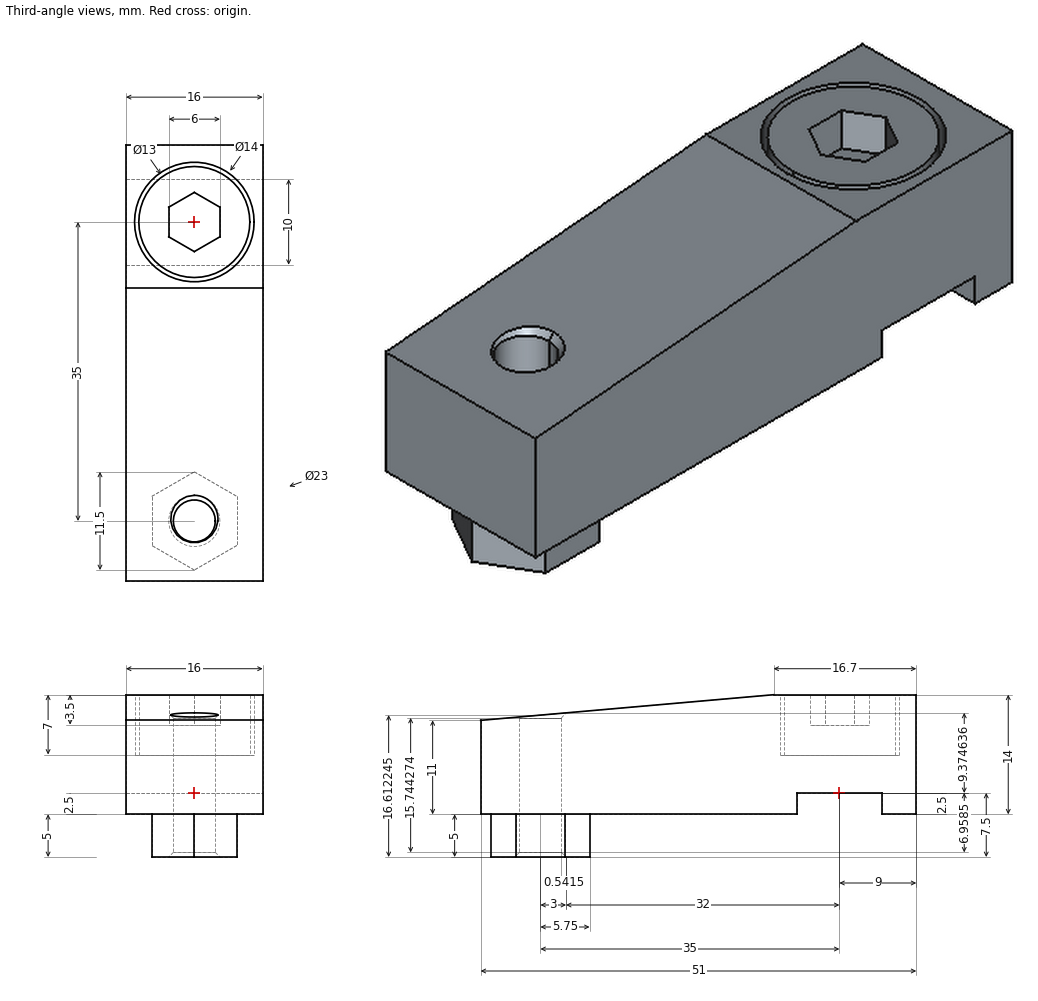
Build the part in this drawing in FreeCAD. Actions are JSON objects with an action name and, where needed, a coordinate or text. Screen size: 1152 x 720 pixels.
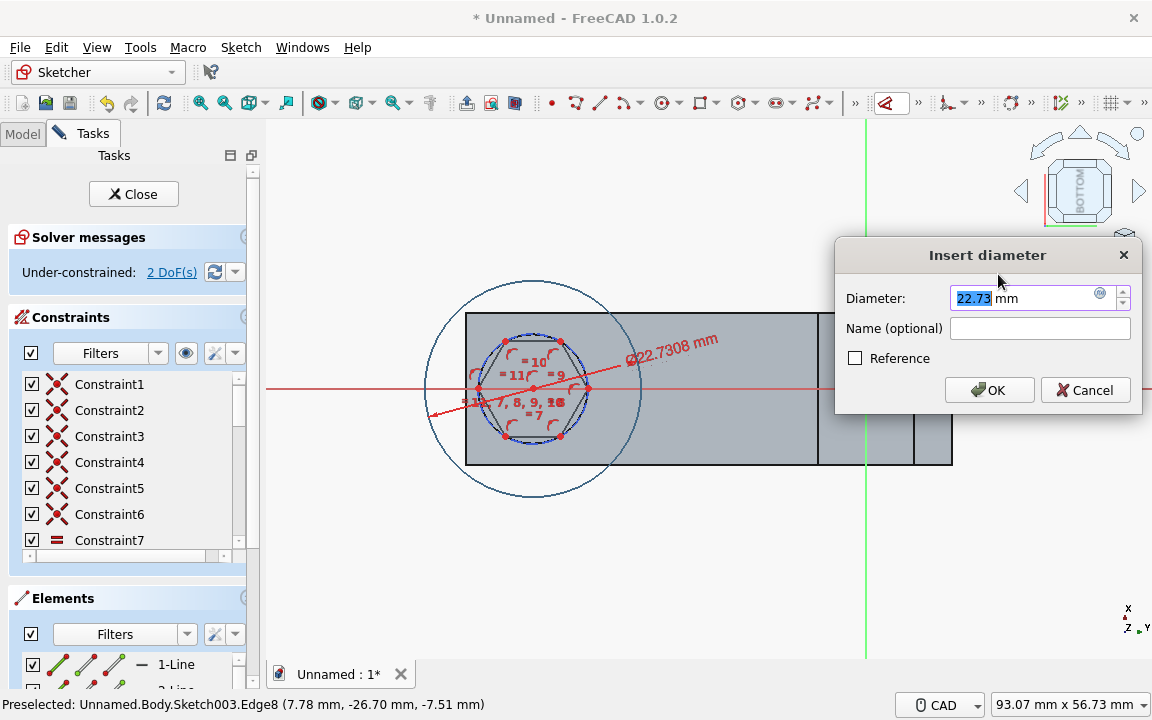
{"action": "type", "text": "23"}
{"action": "key", "text": "Return"}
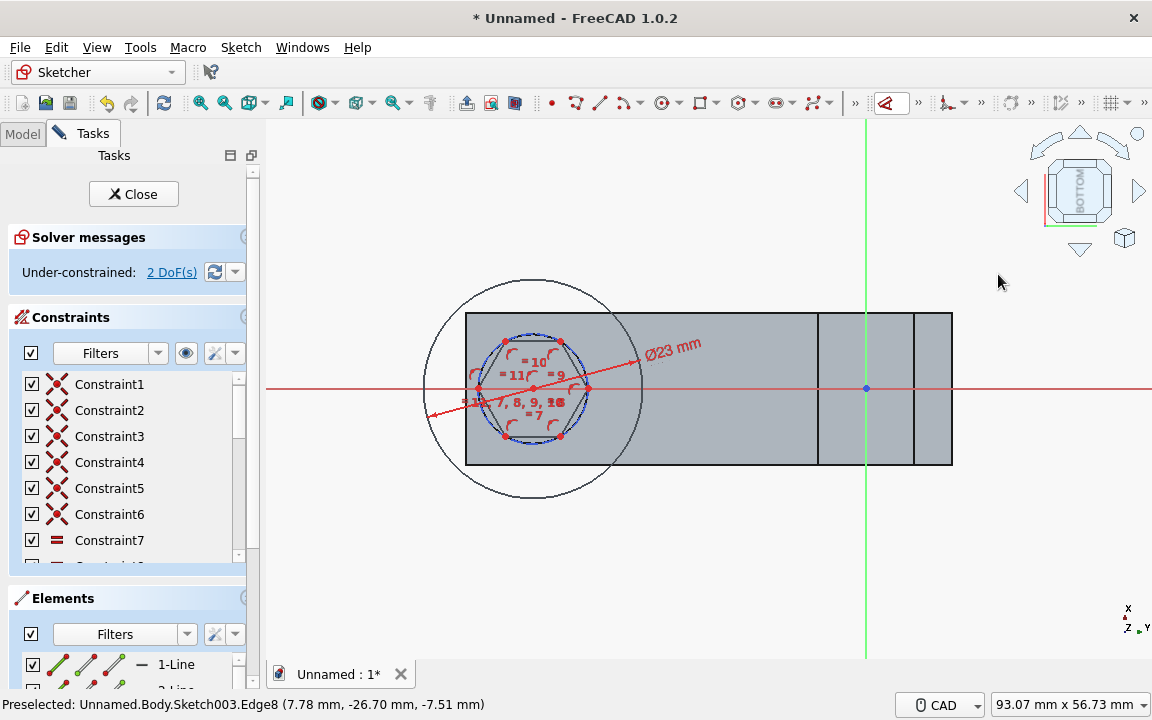
{"action": "left_click", "coordinate": [533, 389]}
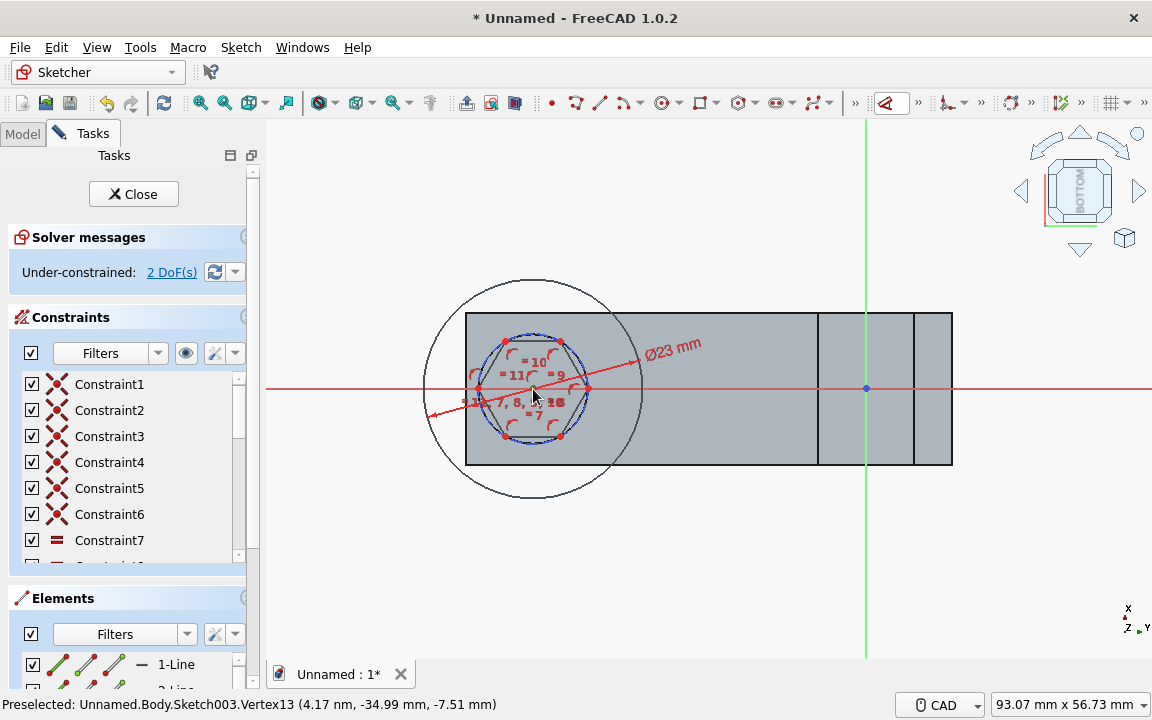
{"action": "left_click", "coordinate": [904, 104]}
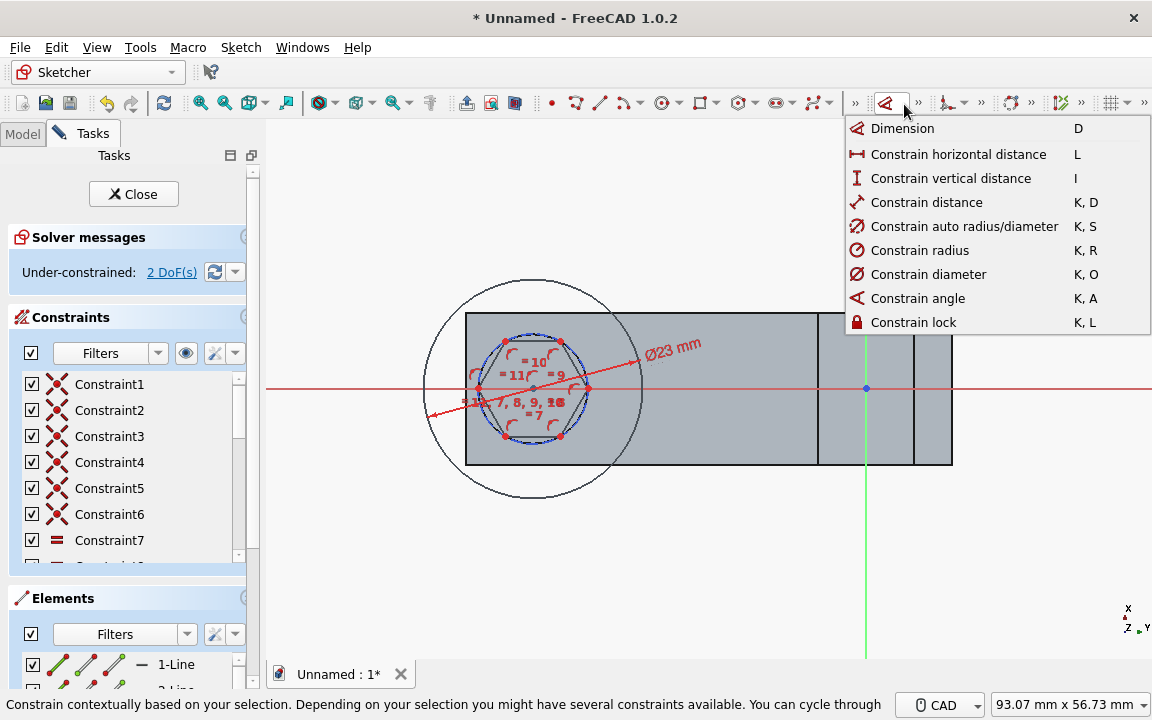
{"action": "left_click", "coordinate": [998, 154]}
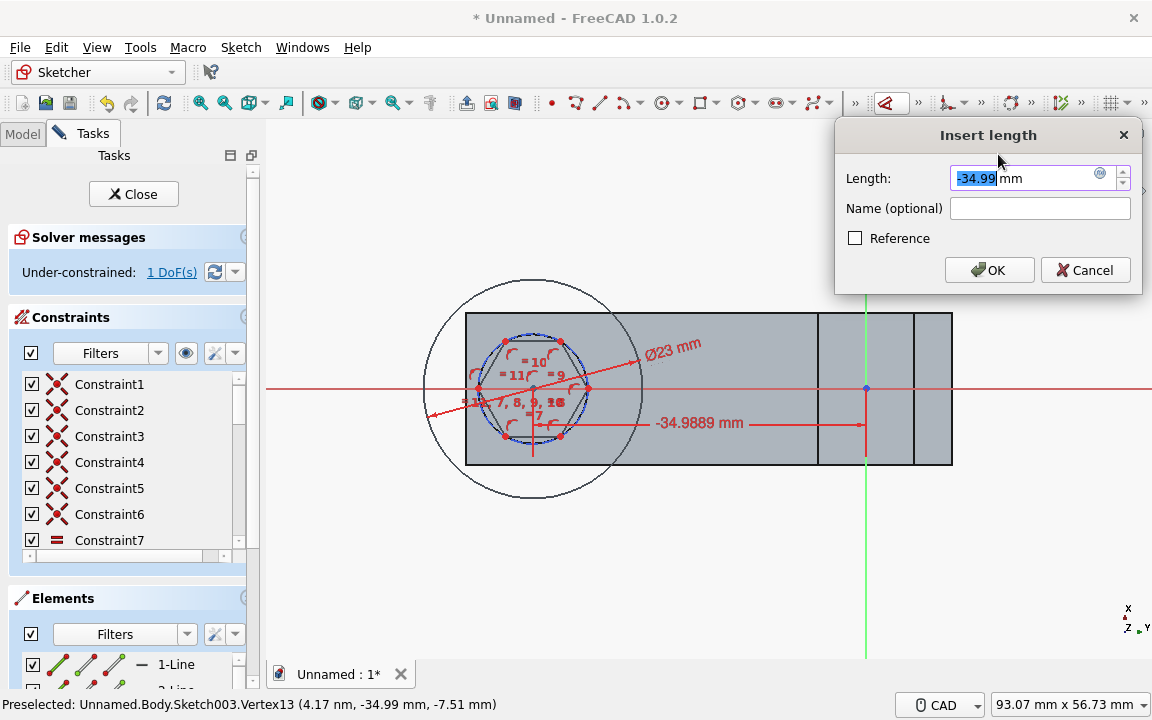
{"action": "type", "text": "-35"}
{"action": "key", "text": "Return"}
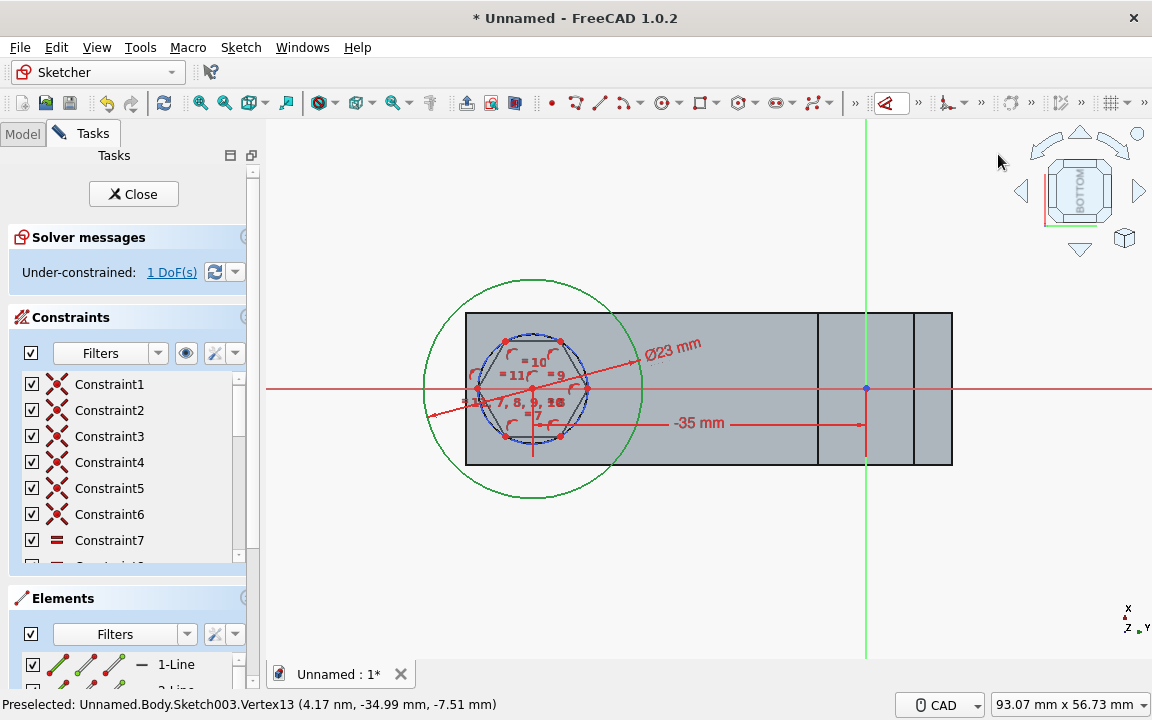
{"action": "left_click", "coordinate": [478, 389]}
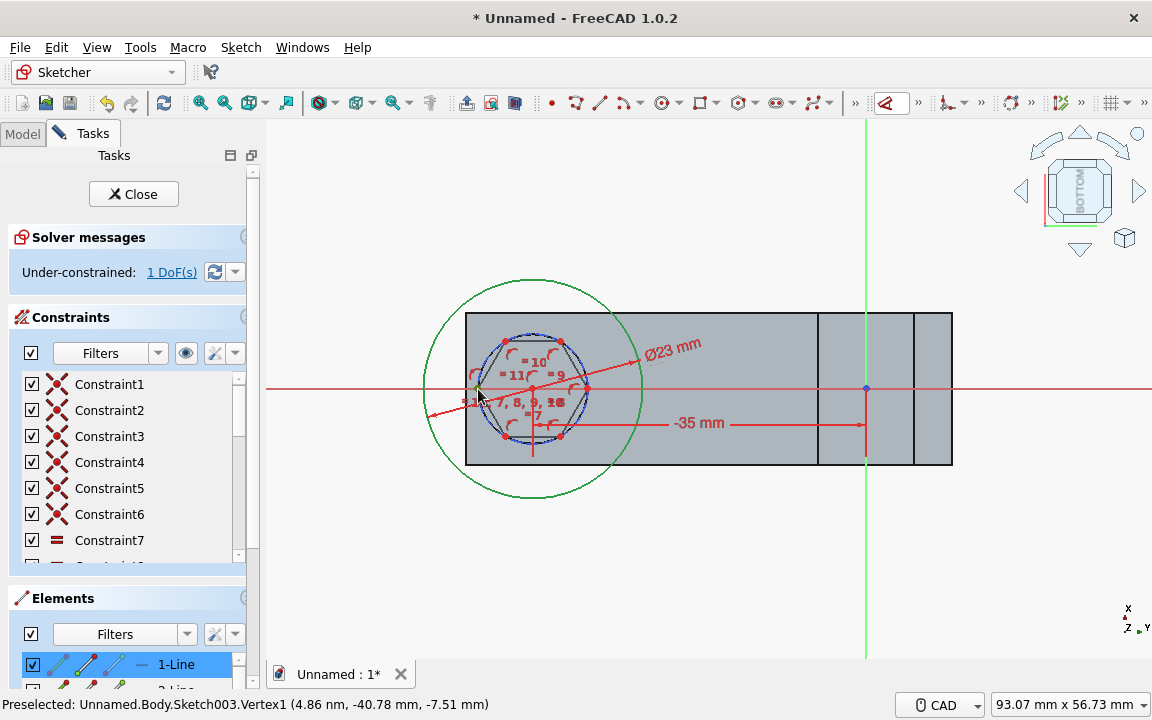
{"action": "left_click", "coordinate": [588, 389]}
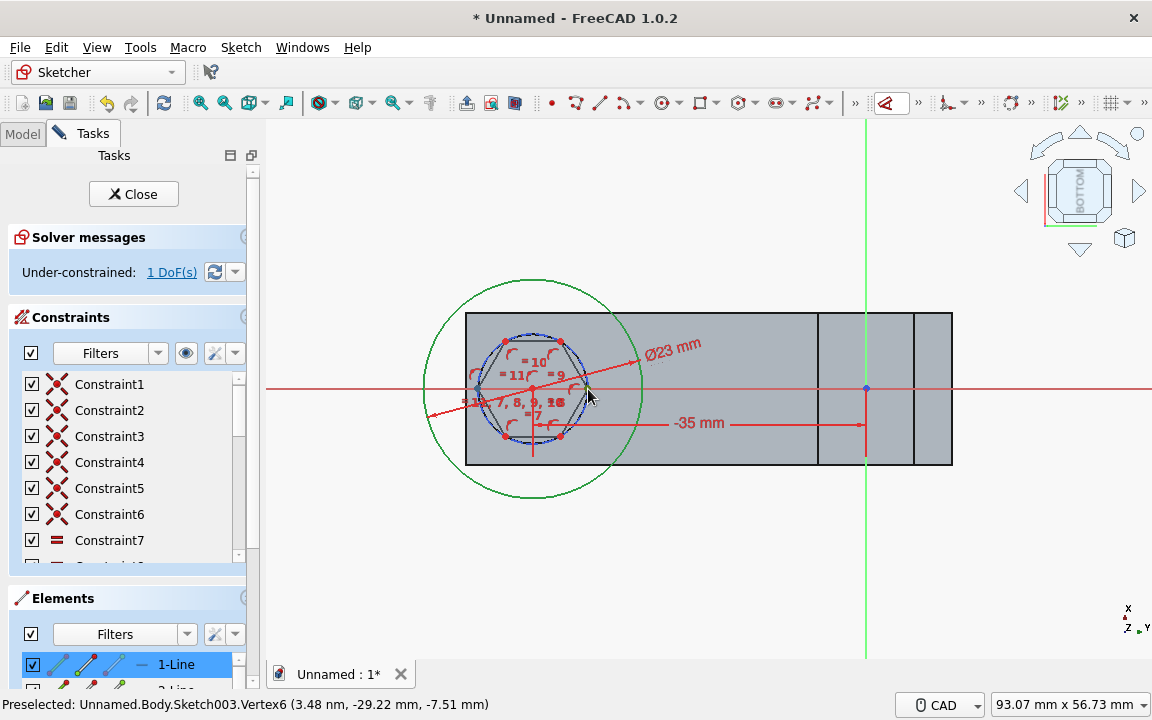
{"action": "left_click", "coordinate": [904, 104]}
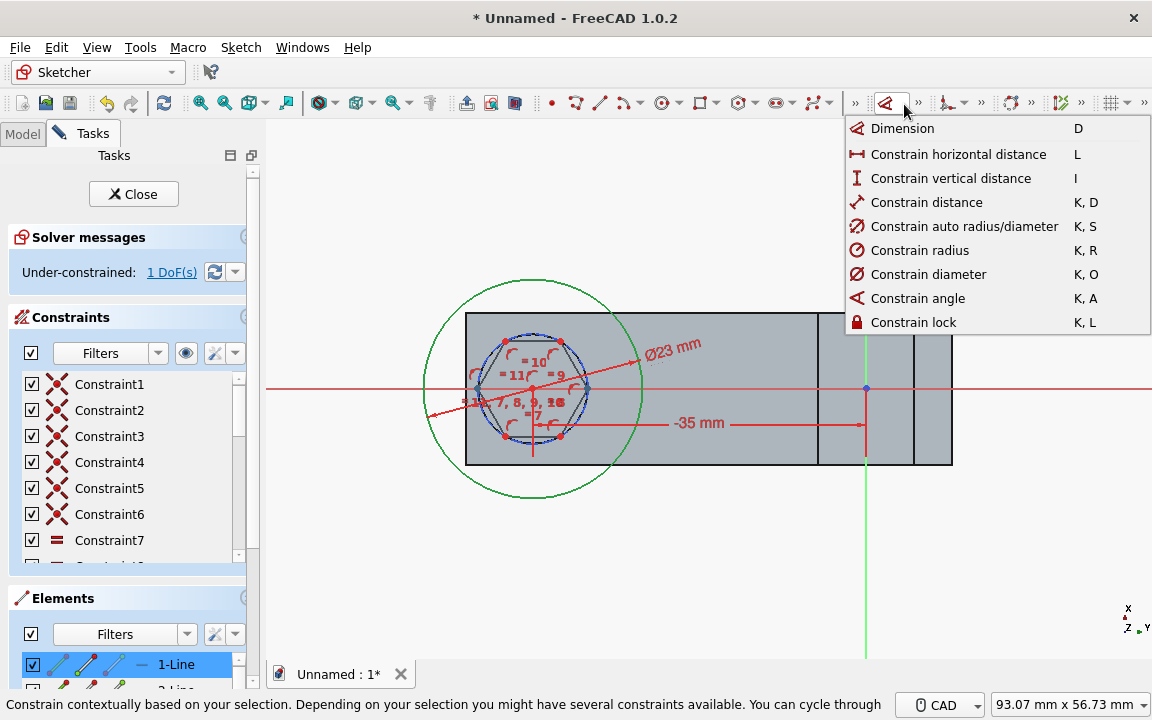
{"action": "left_click", "coordinate": [998, 154]}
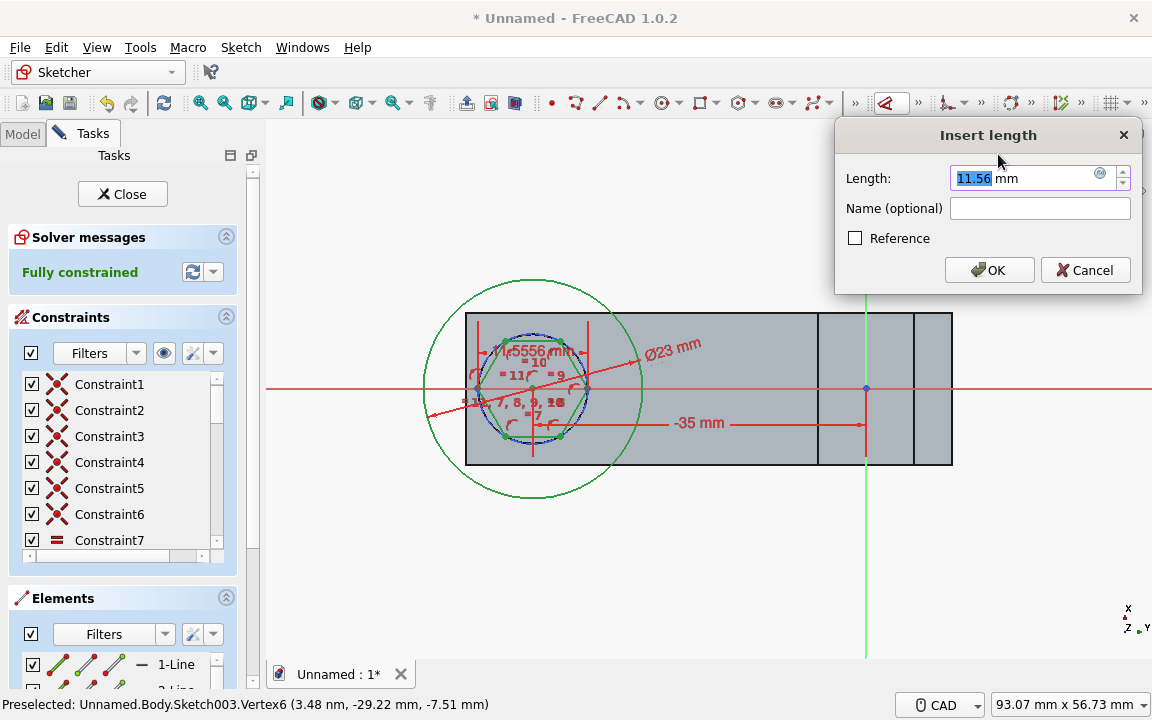
{"action": "type", "text": "11.5"}
{"action": "key", "text": "Return"}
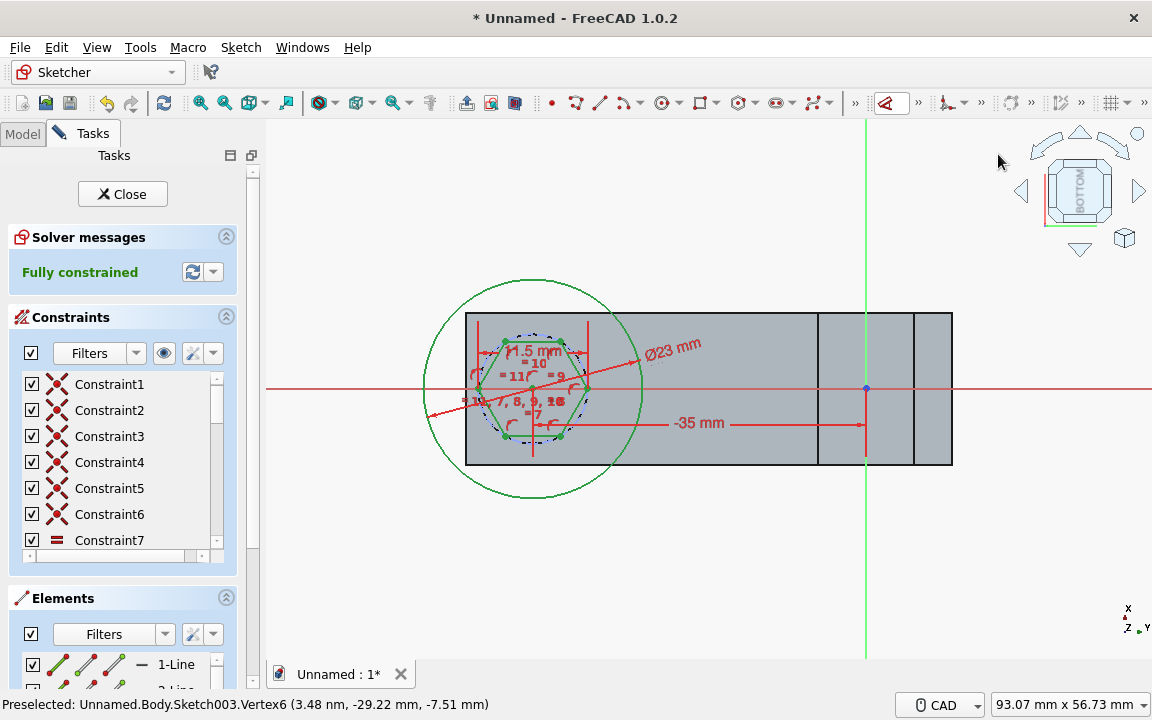
{"action": "left_click", "coordinate": [123, 194]}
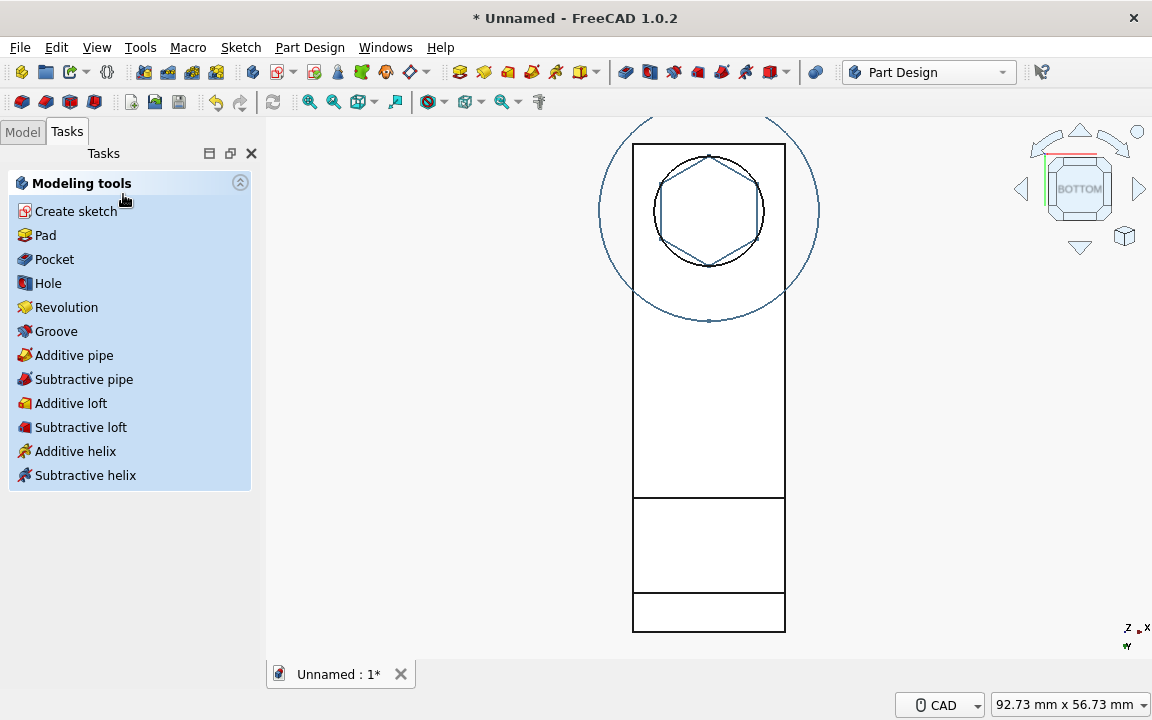
{"action": "left_click", "coordinate": [626, 72]}